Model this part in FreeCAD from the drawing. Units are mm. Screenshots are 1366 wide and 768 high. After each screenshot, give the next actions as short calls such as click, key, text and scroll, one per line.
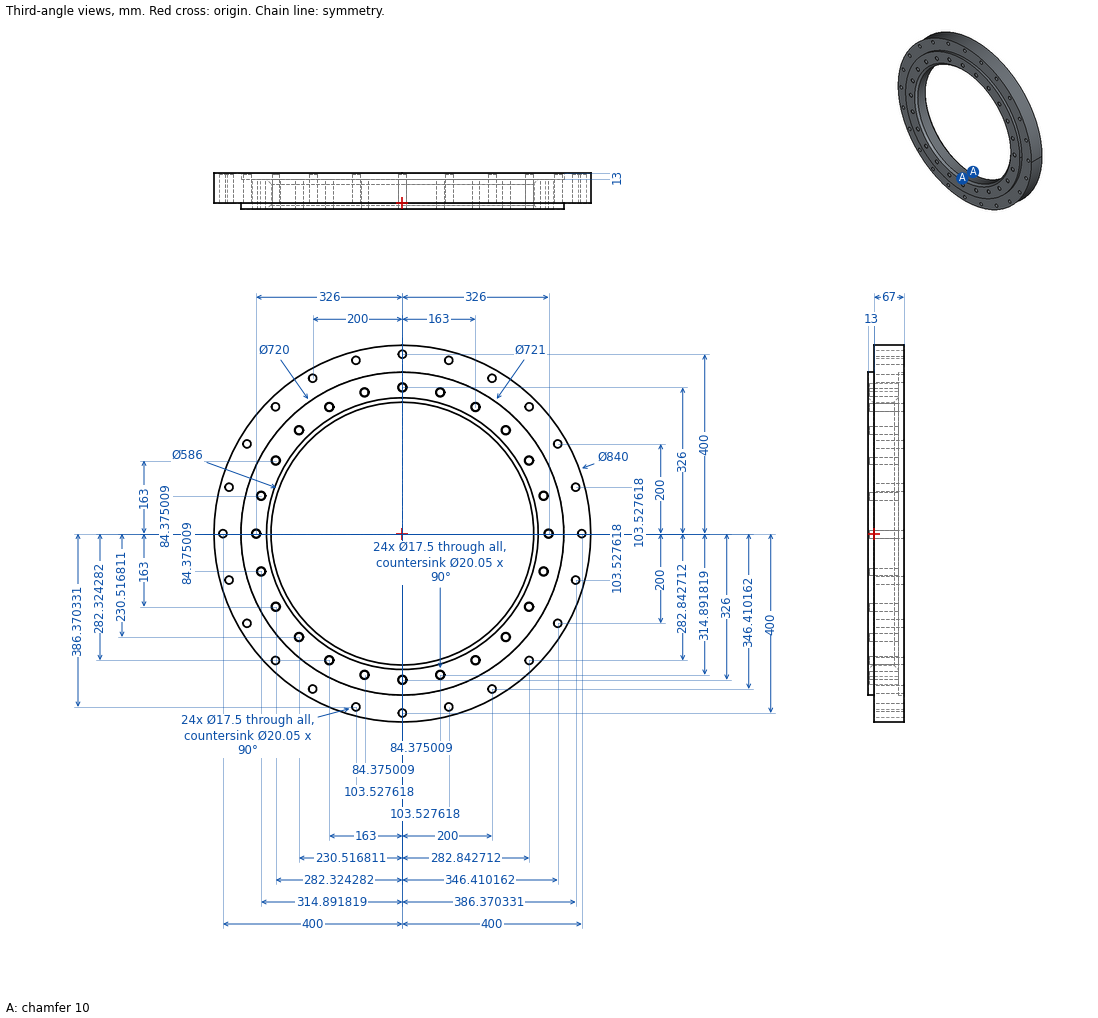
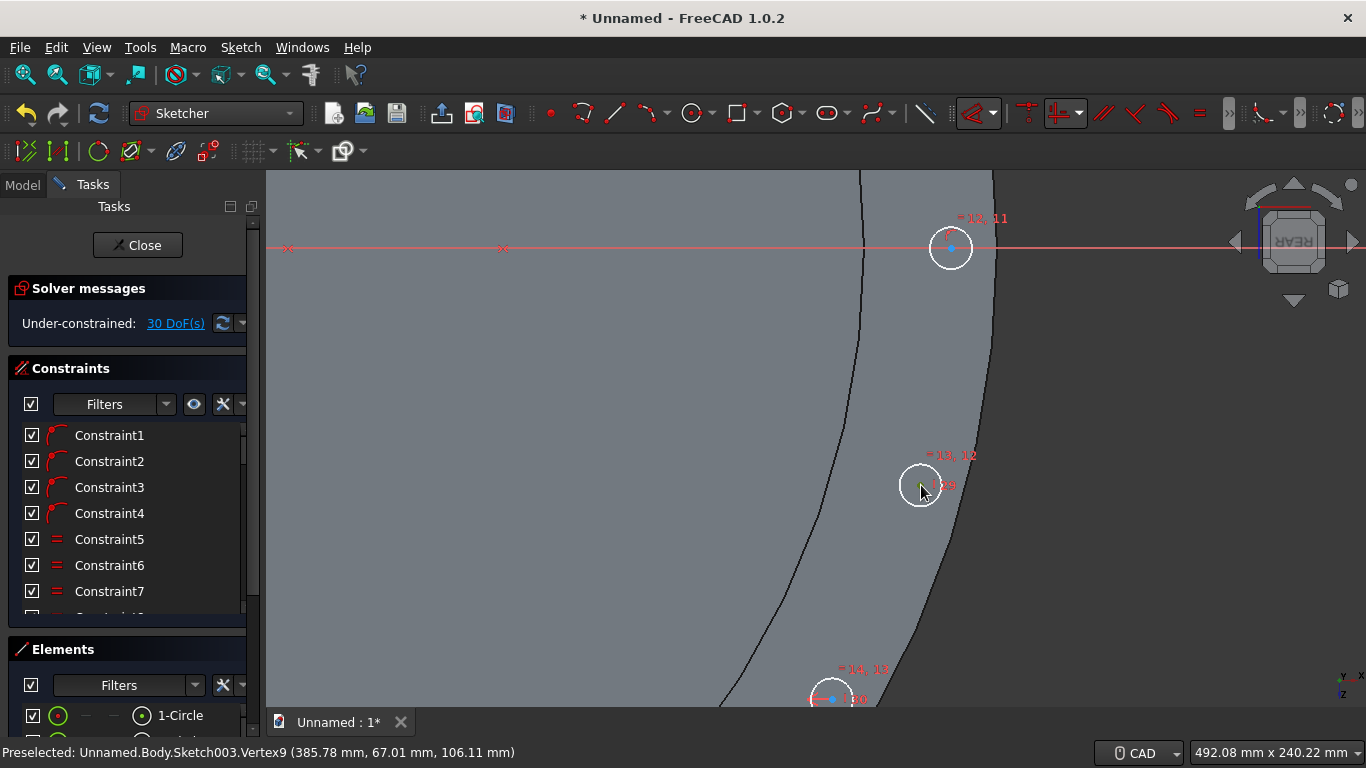
scroll(922, 487, down, 8)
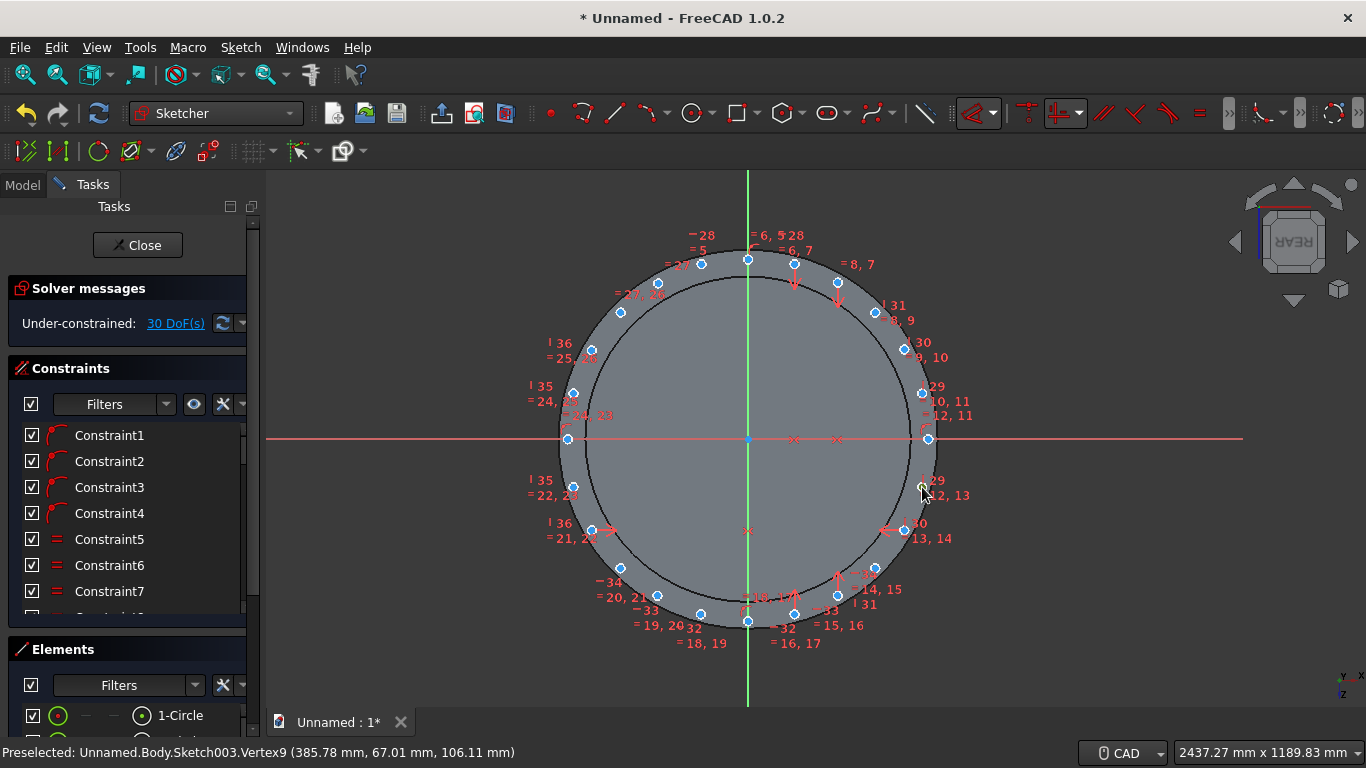
click(573, 487)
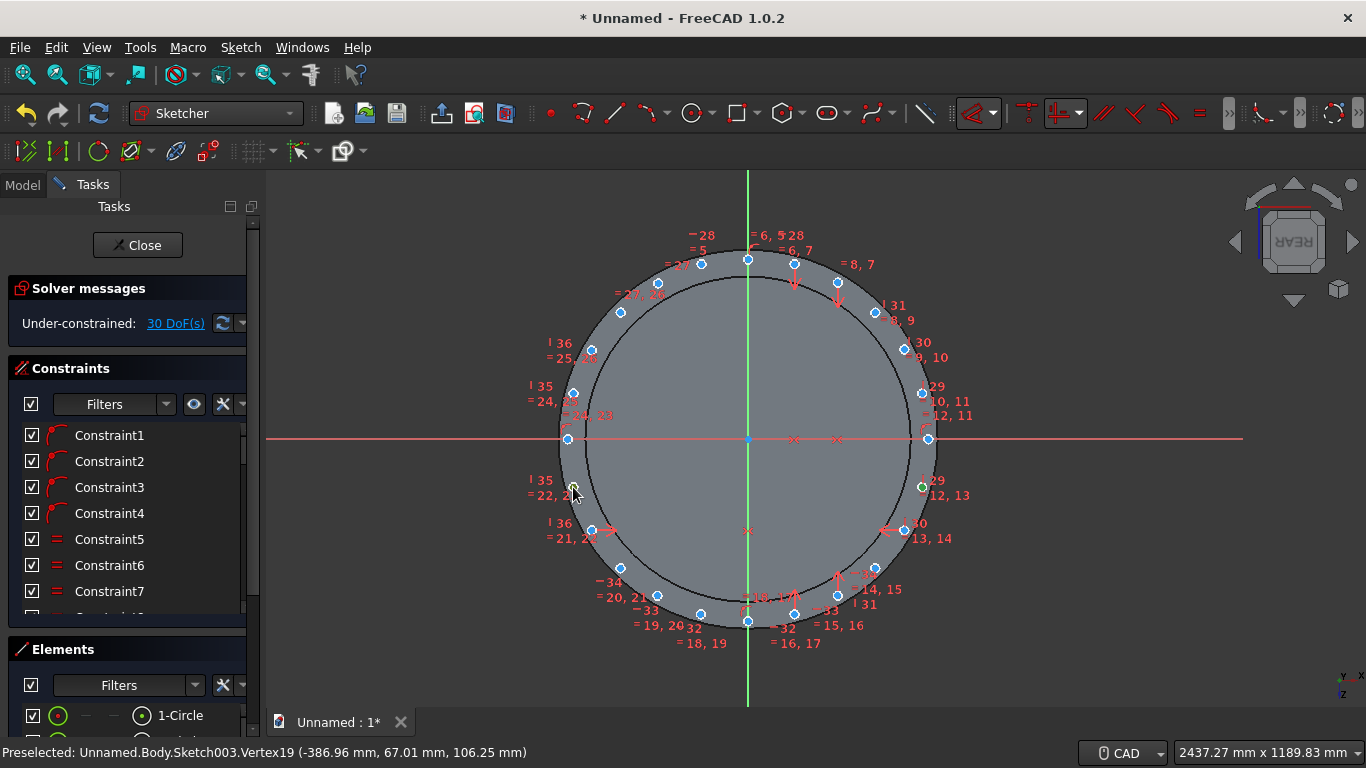
click(748, 576)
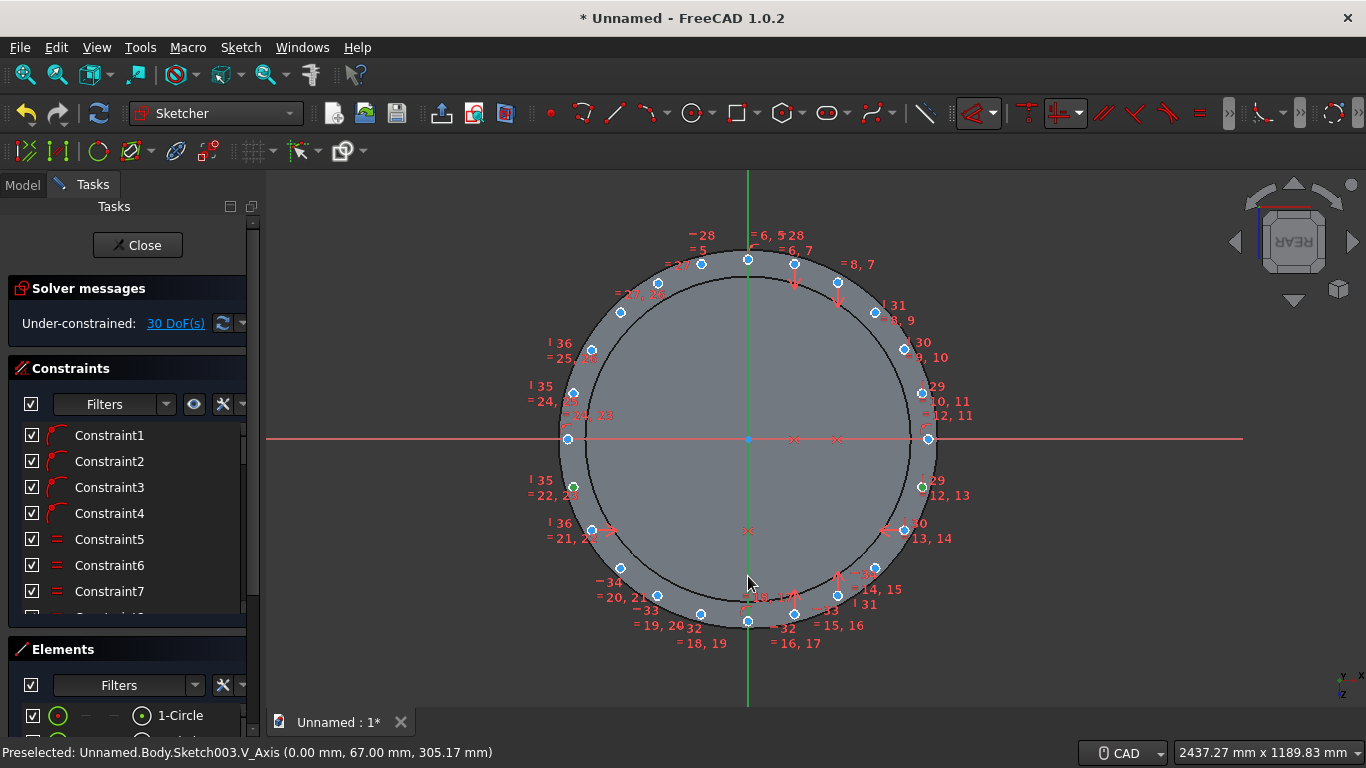
key(s)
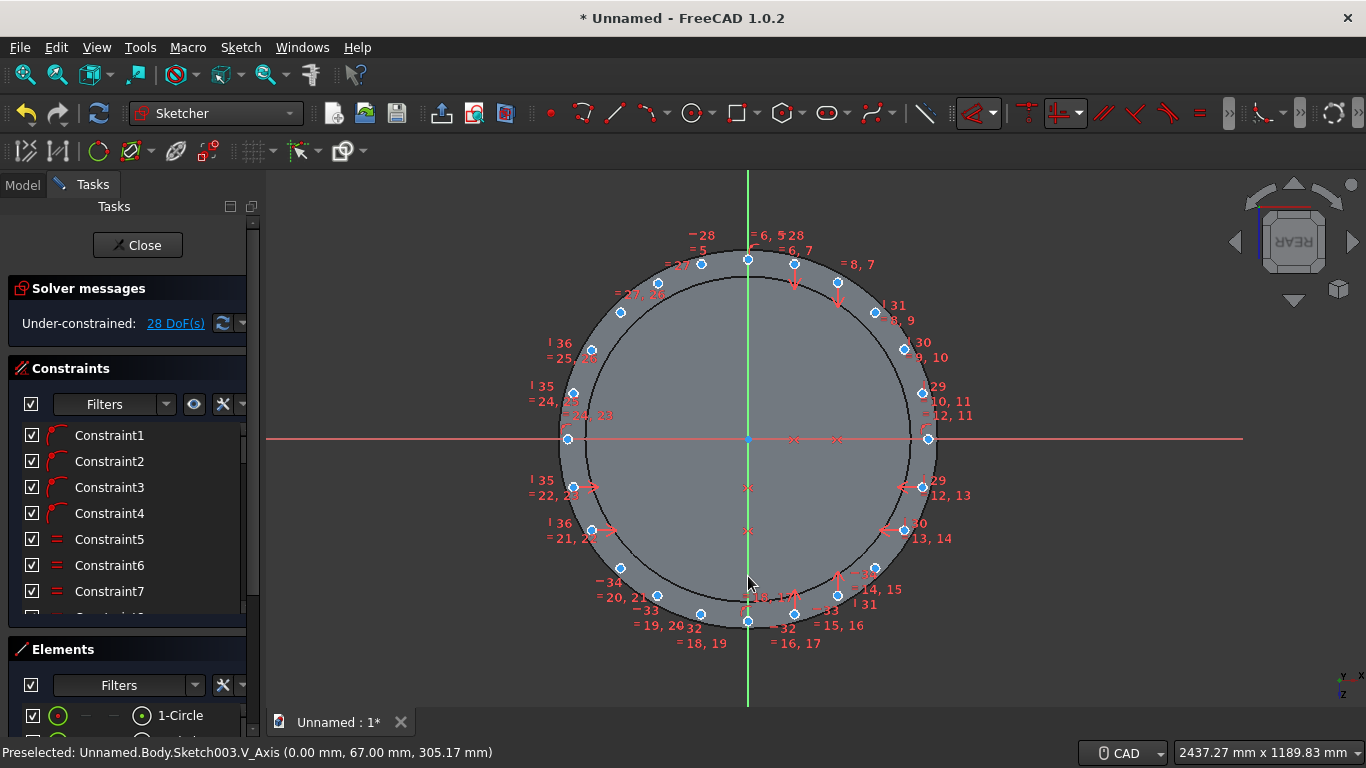
click(875, 313)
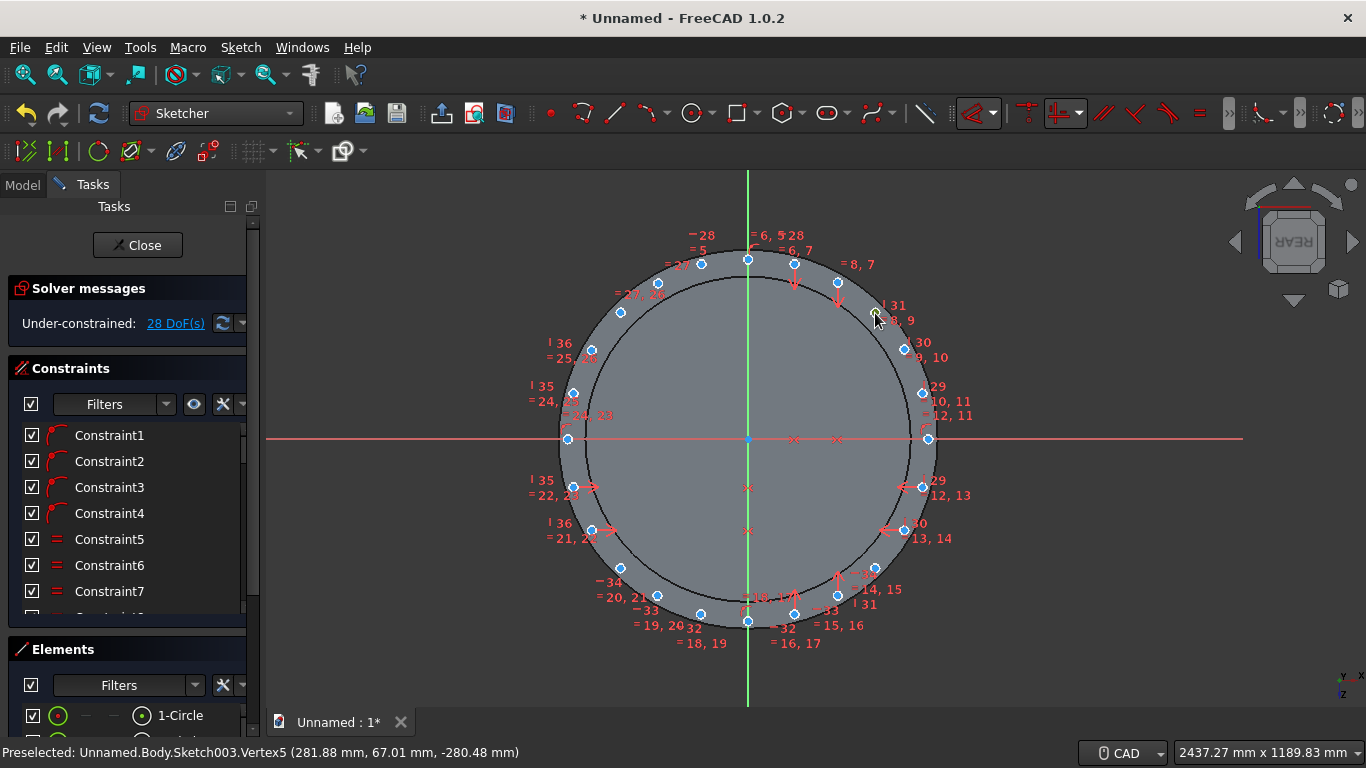
click(621, 313)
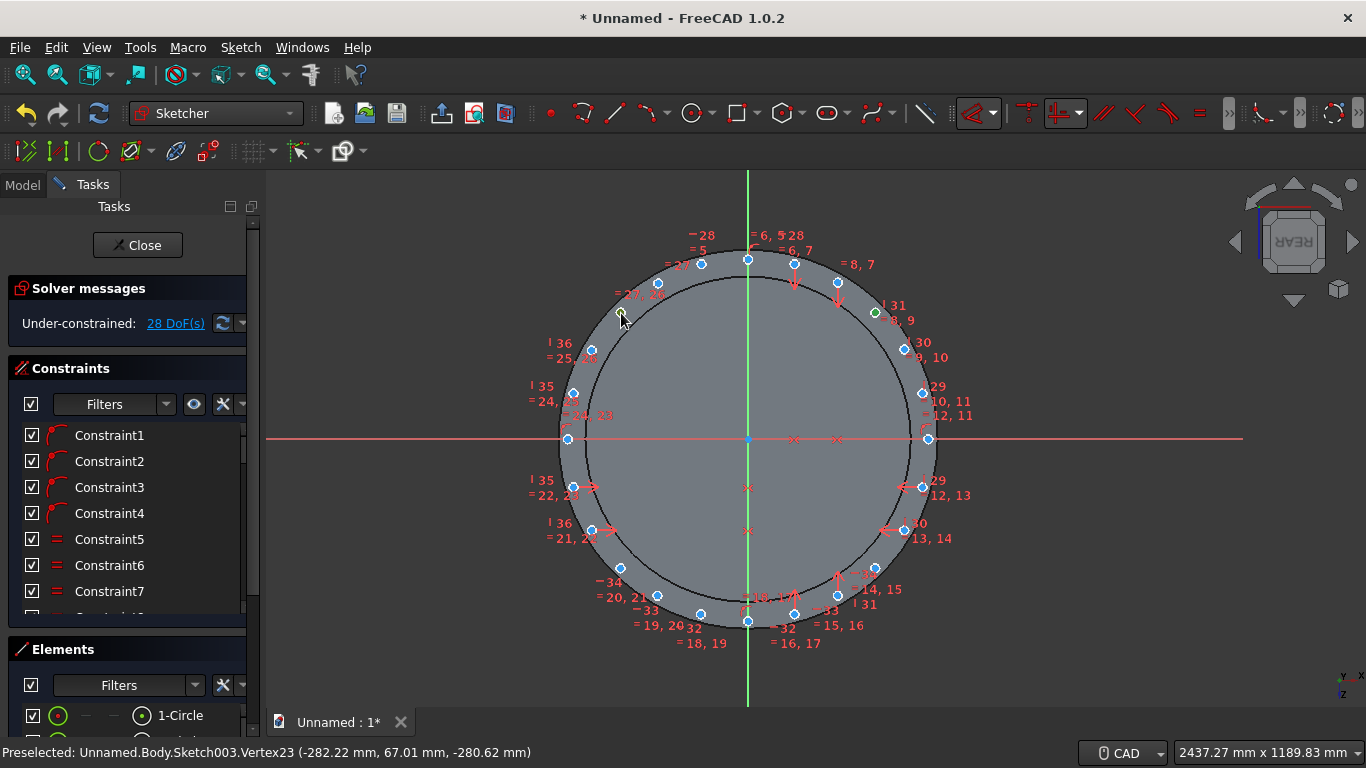
click(748, 576)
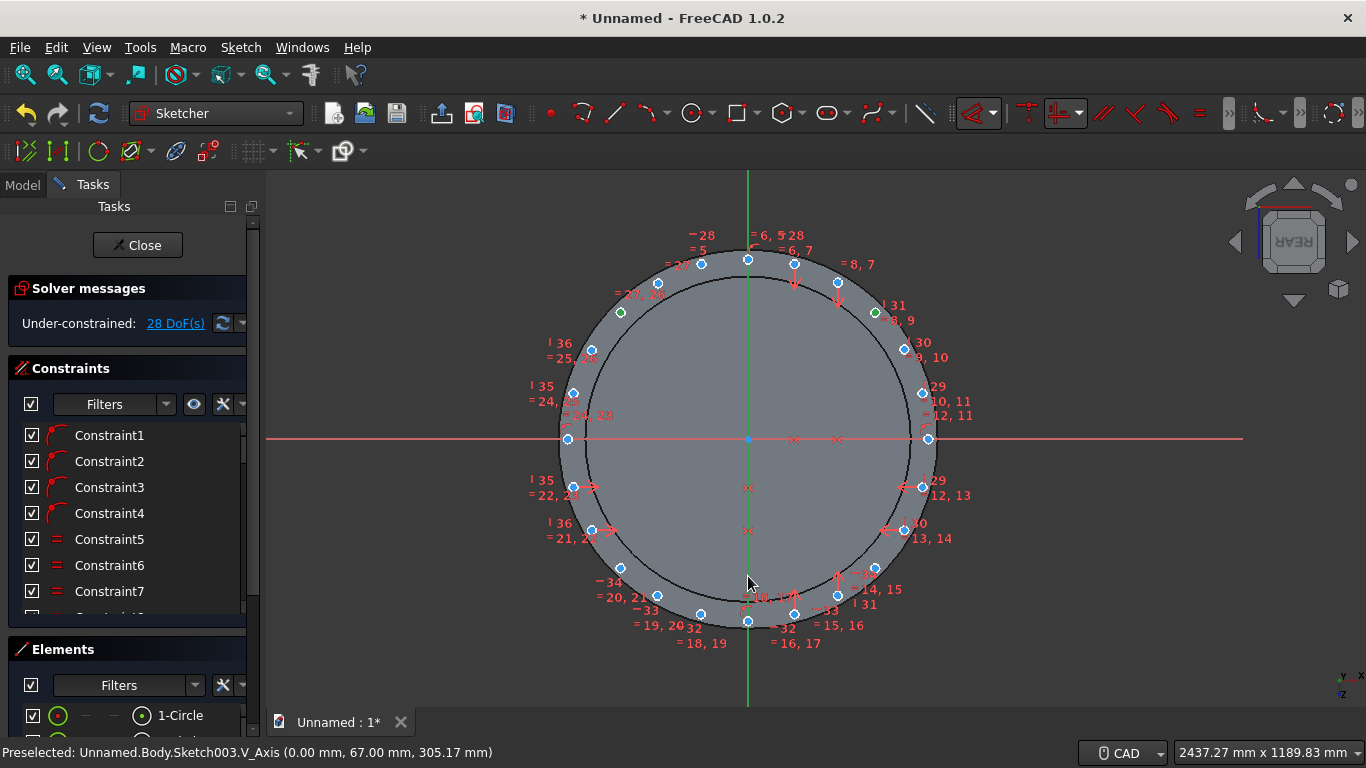
key(s)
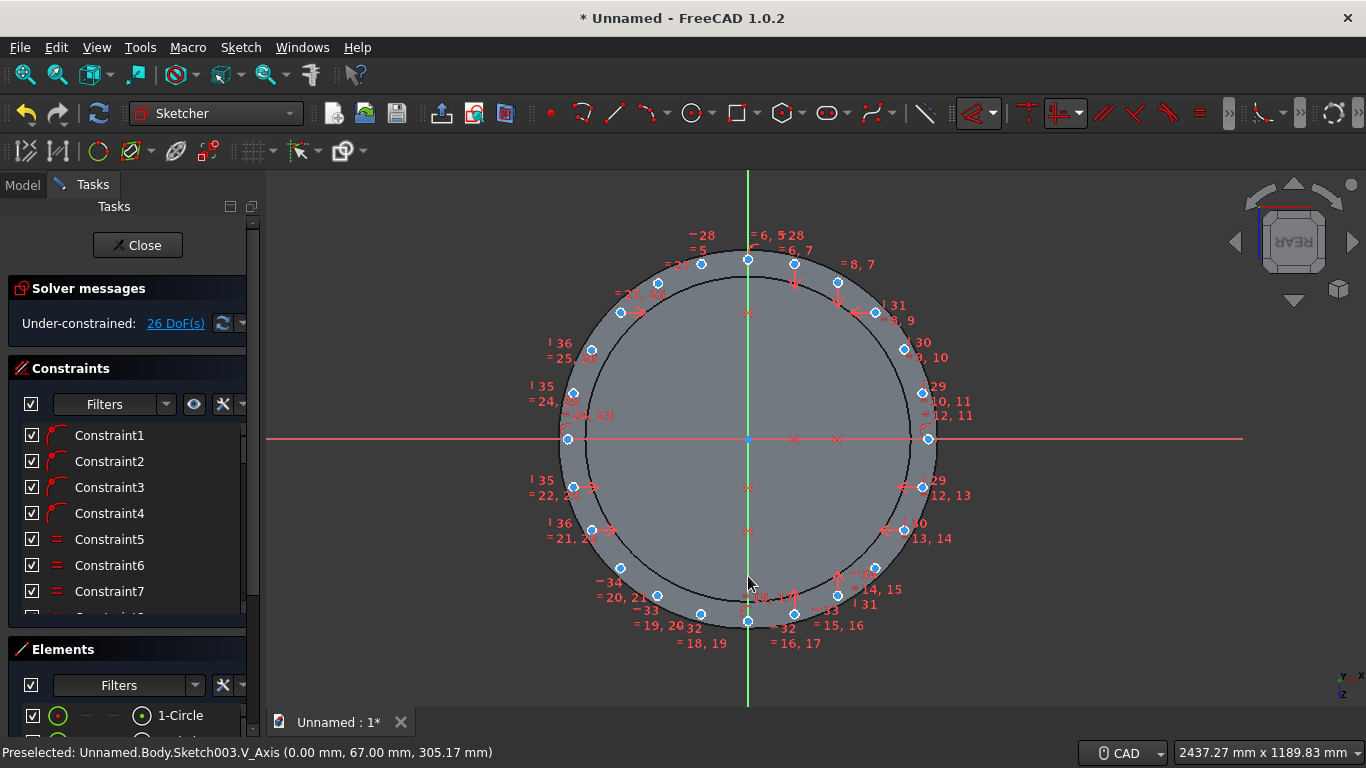
click(621, 568)